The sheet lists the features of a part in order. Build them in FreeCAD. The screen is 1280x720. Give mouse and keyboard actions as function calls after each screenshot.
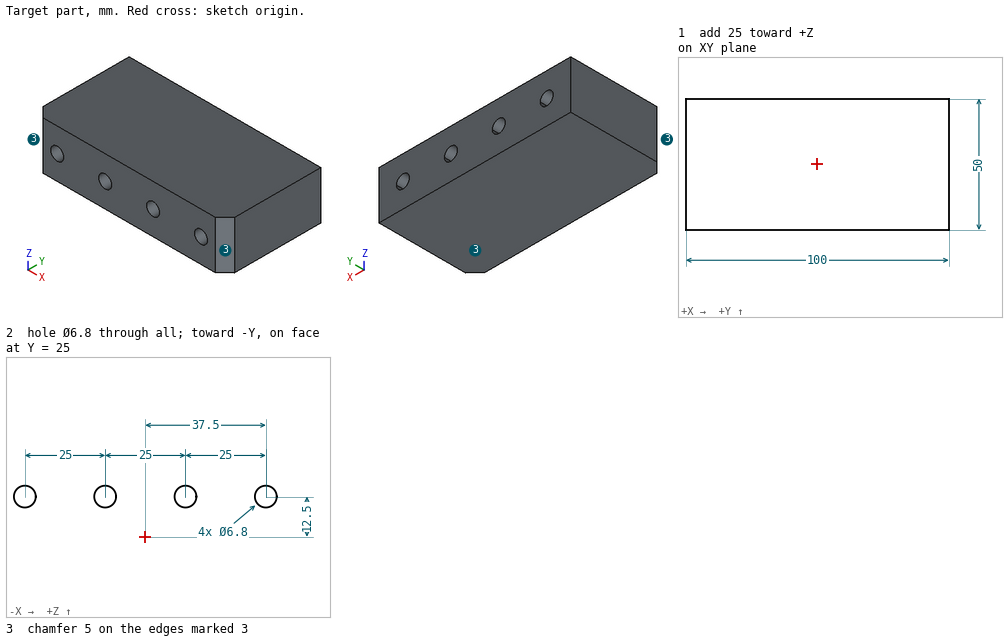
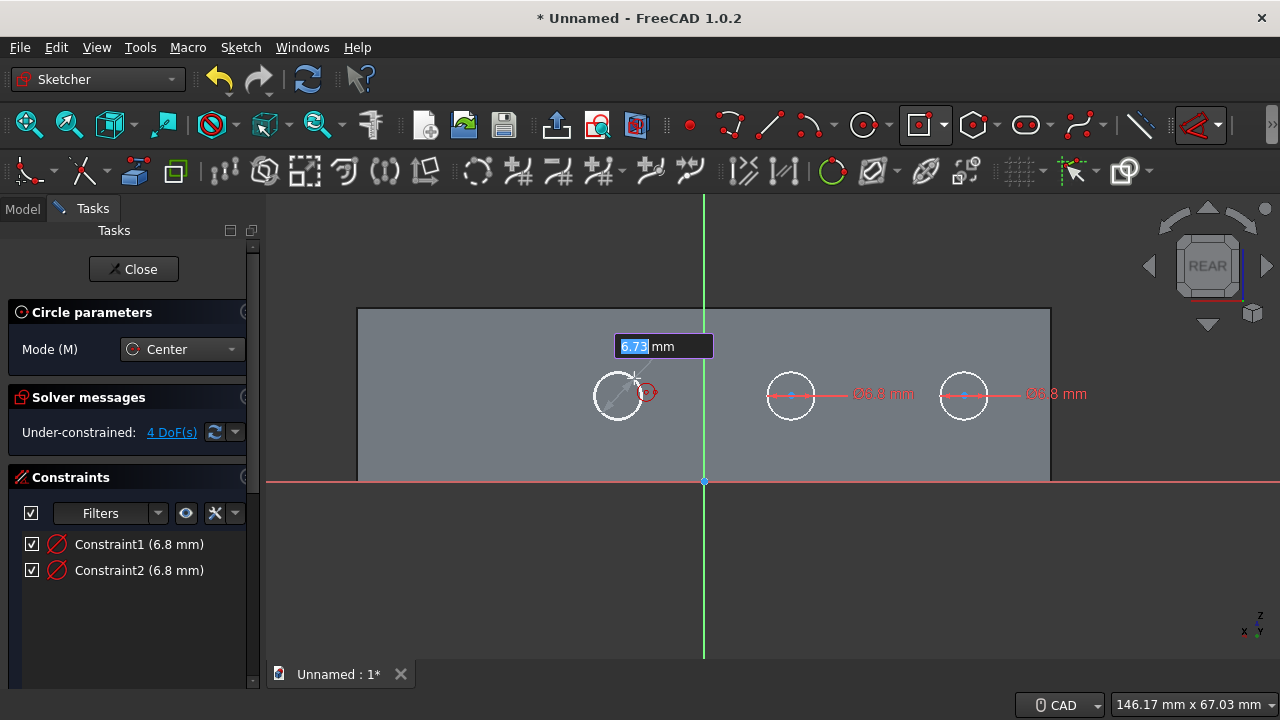
text(6.8)
key(Return)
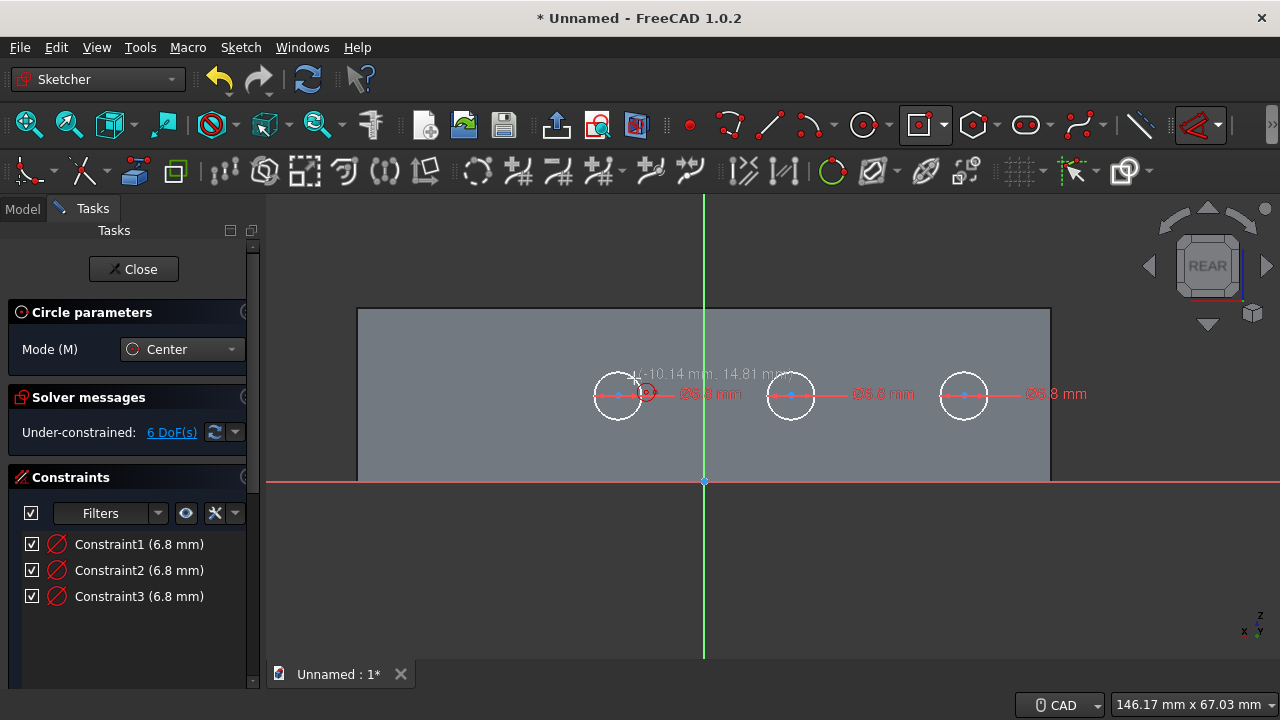
click(444, 395)
move(461, 378)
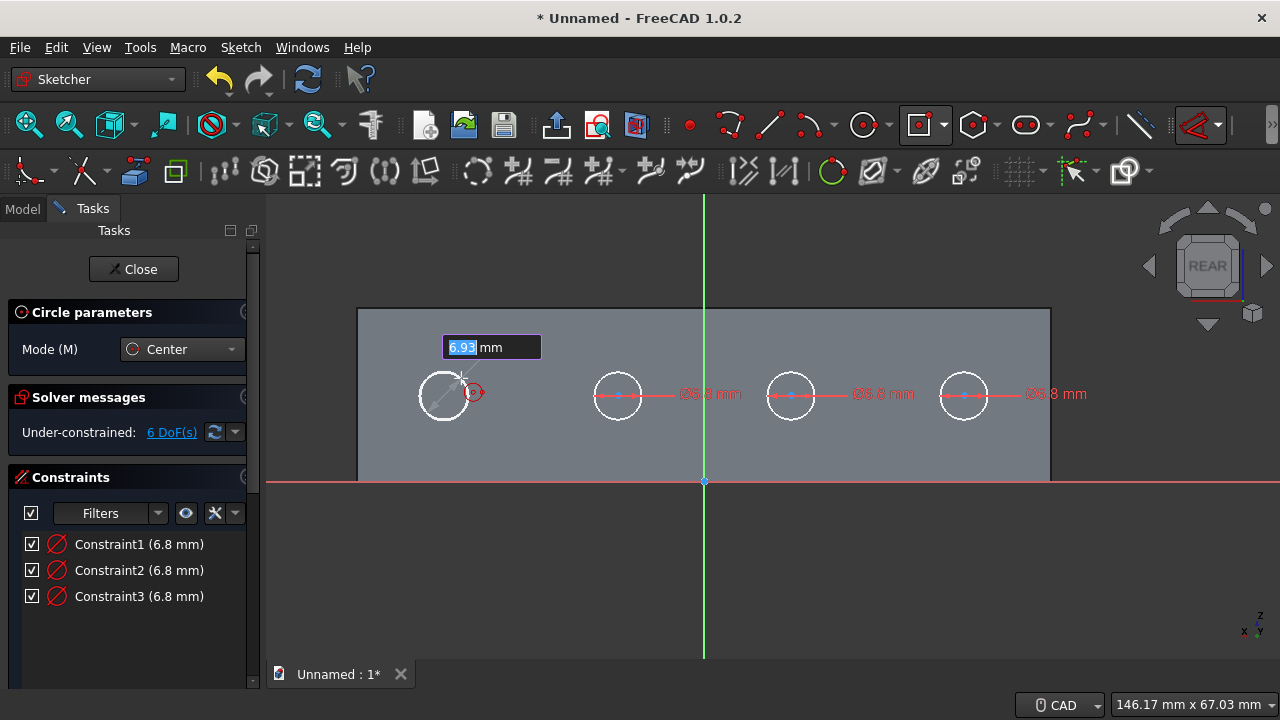
text(6.8)
key(Return)
key(Escape)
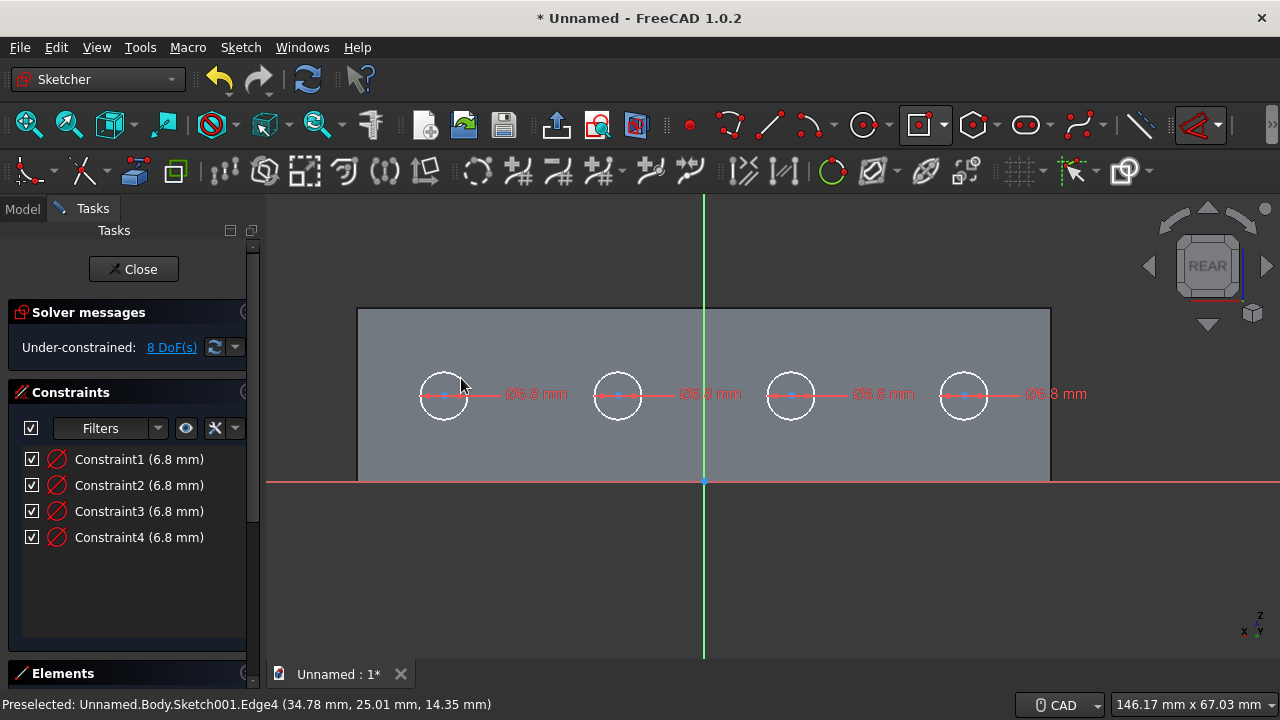
click(964, 396)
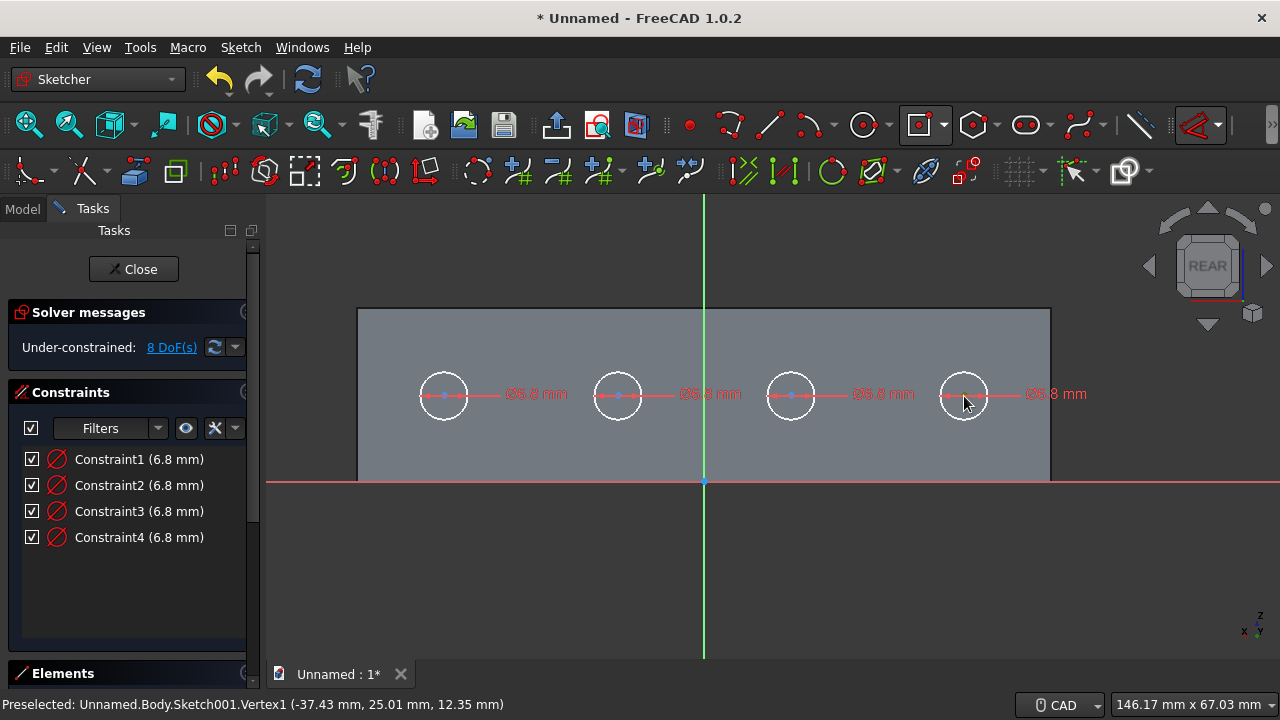
click(791, 396)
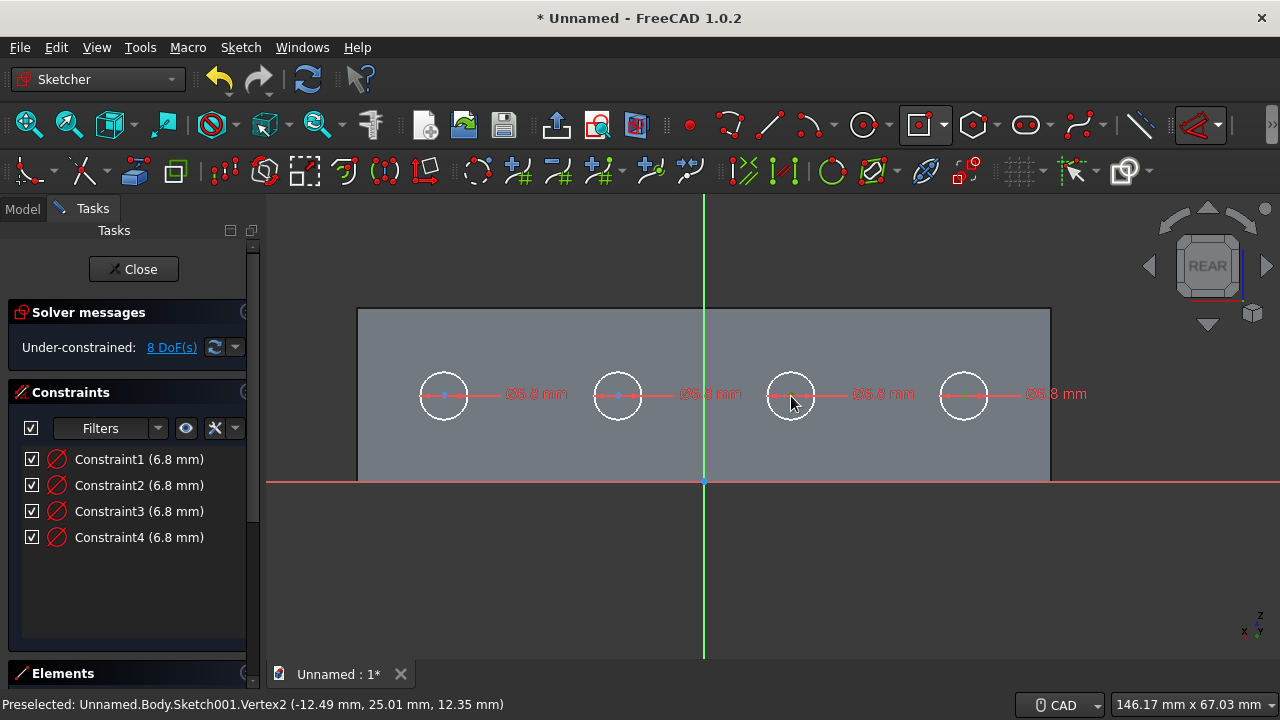
key(h)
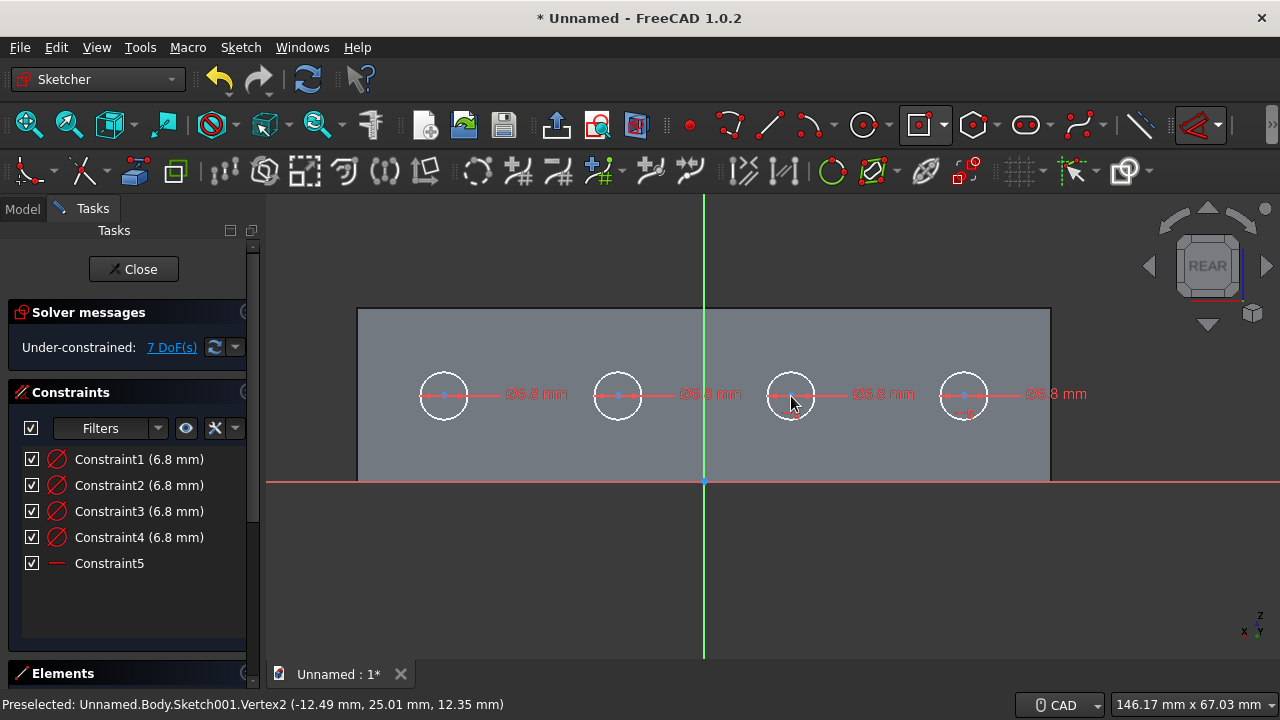
click(791, 396)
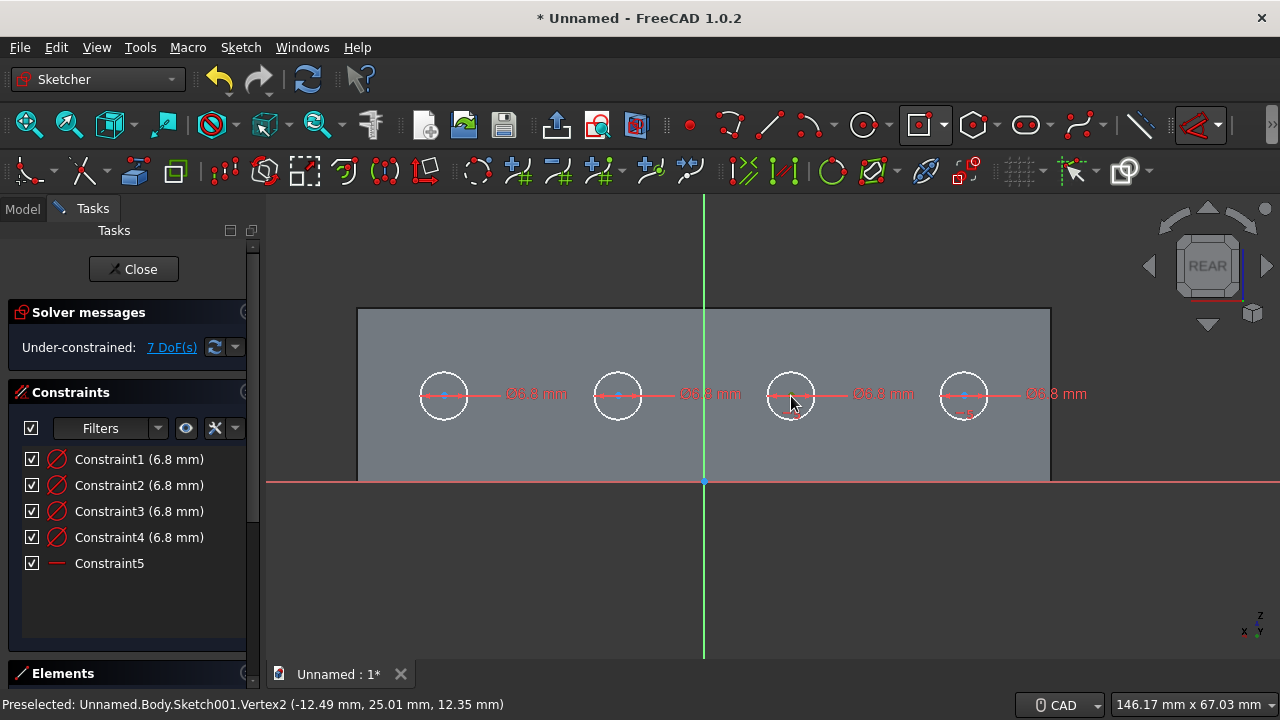
click(618, 396)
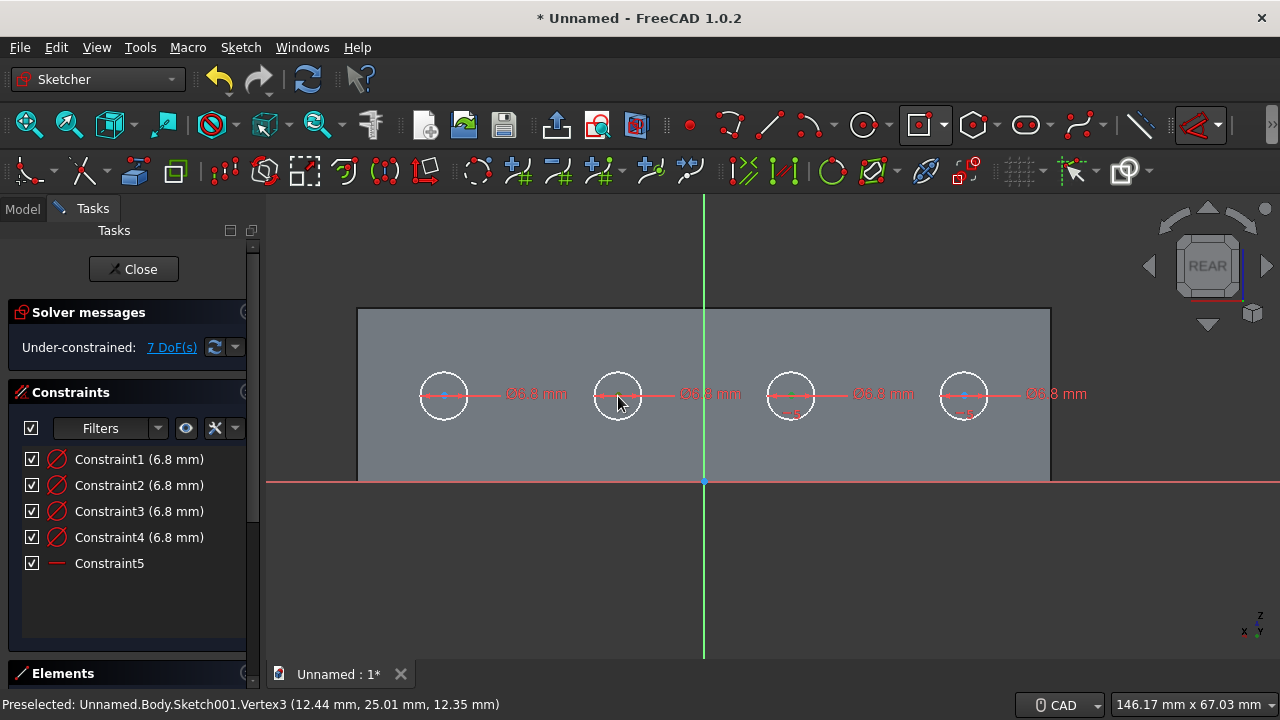
key(h)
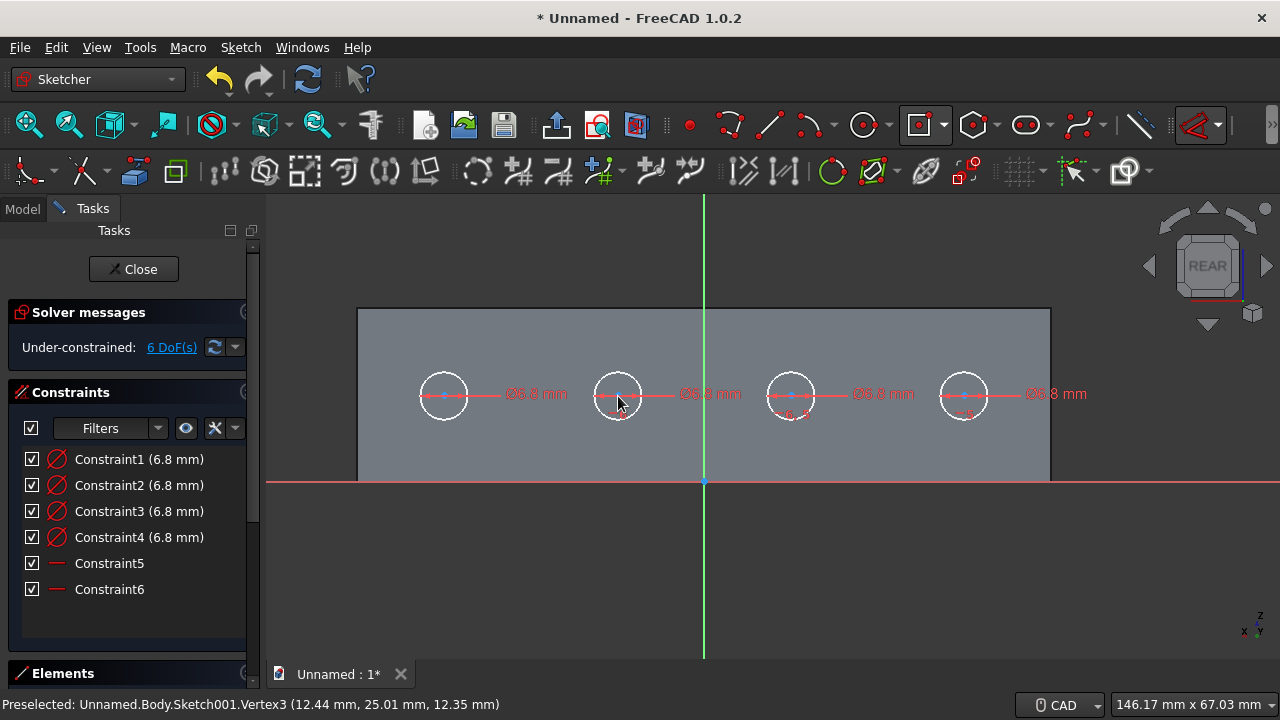
click(618, 396)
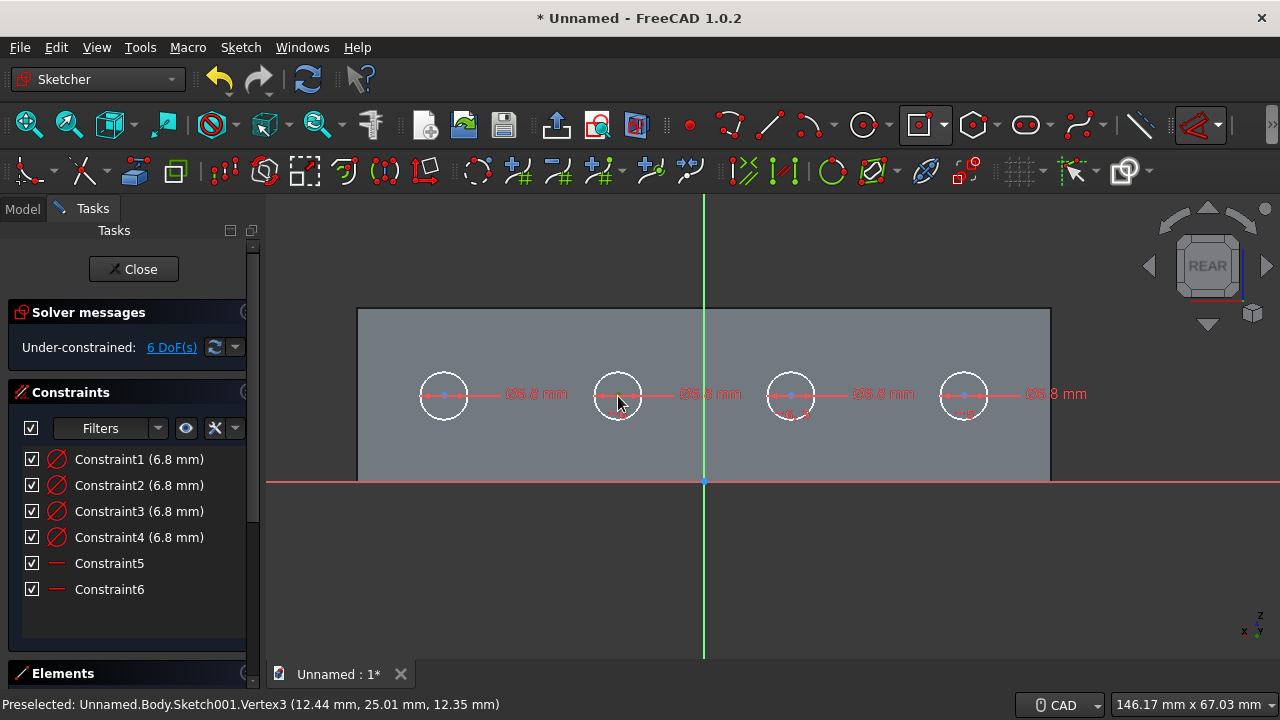
click(444, 396)